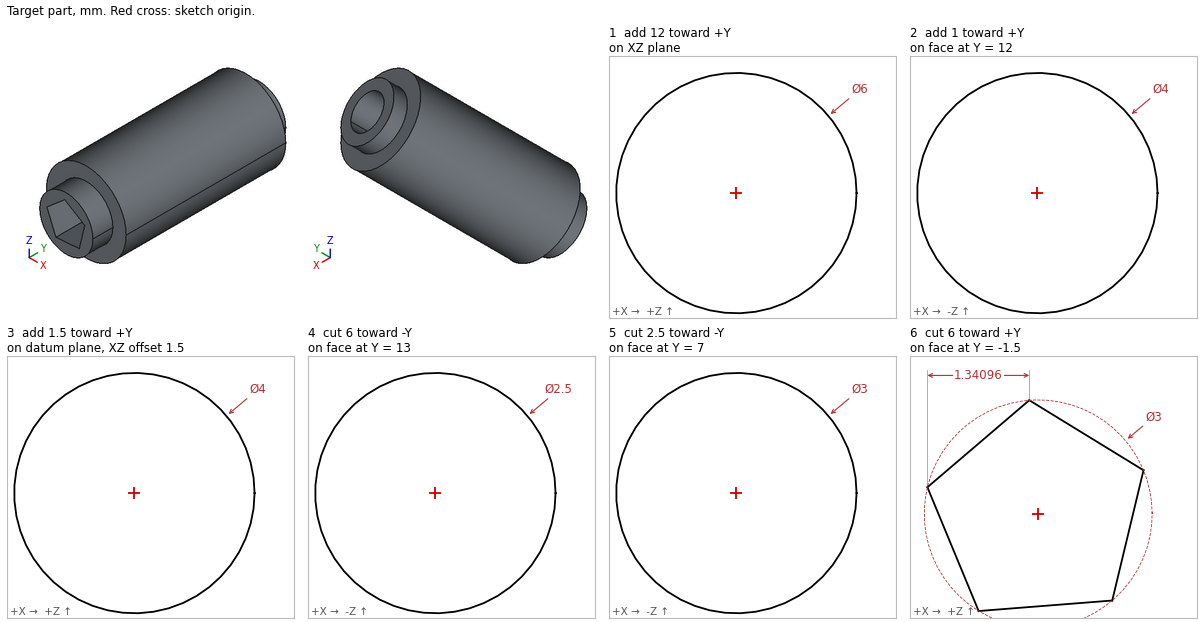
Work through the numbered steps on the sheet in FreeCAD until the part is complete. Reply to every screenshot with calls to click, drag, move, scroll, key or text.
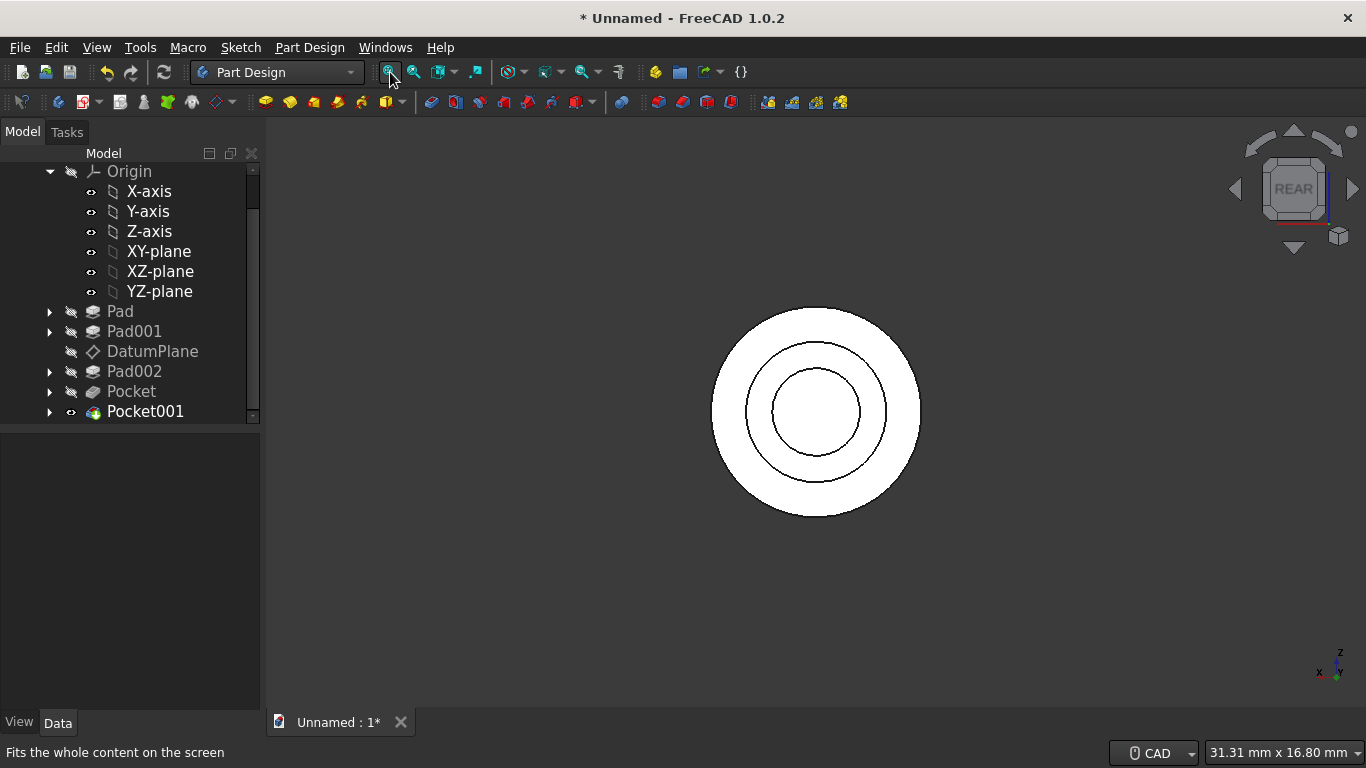
key(0)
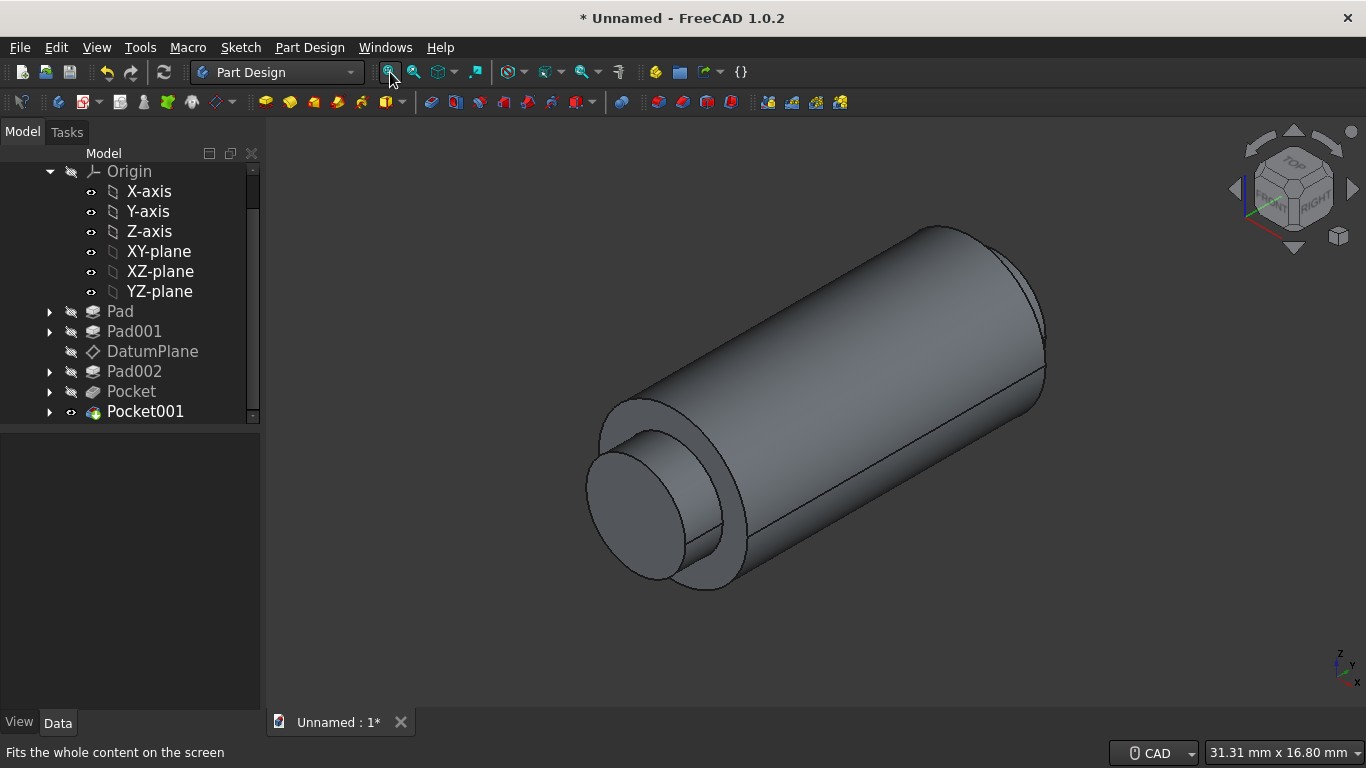
click(636, 515)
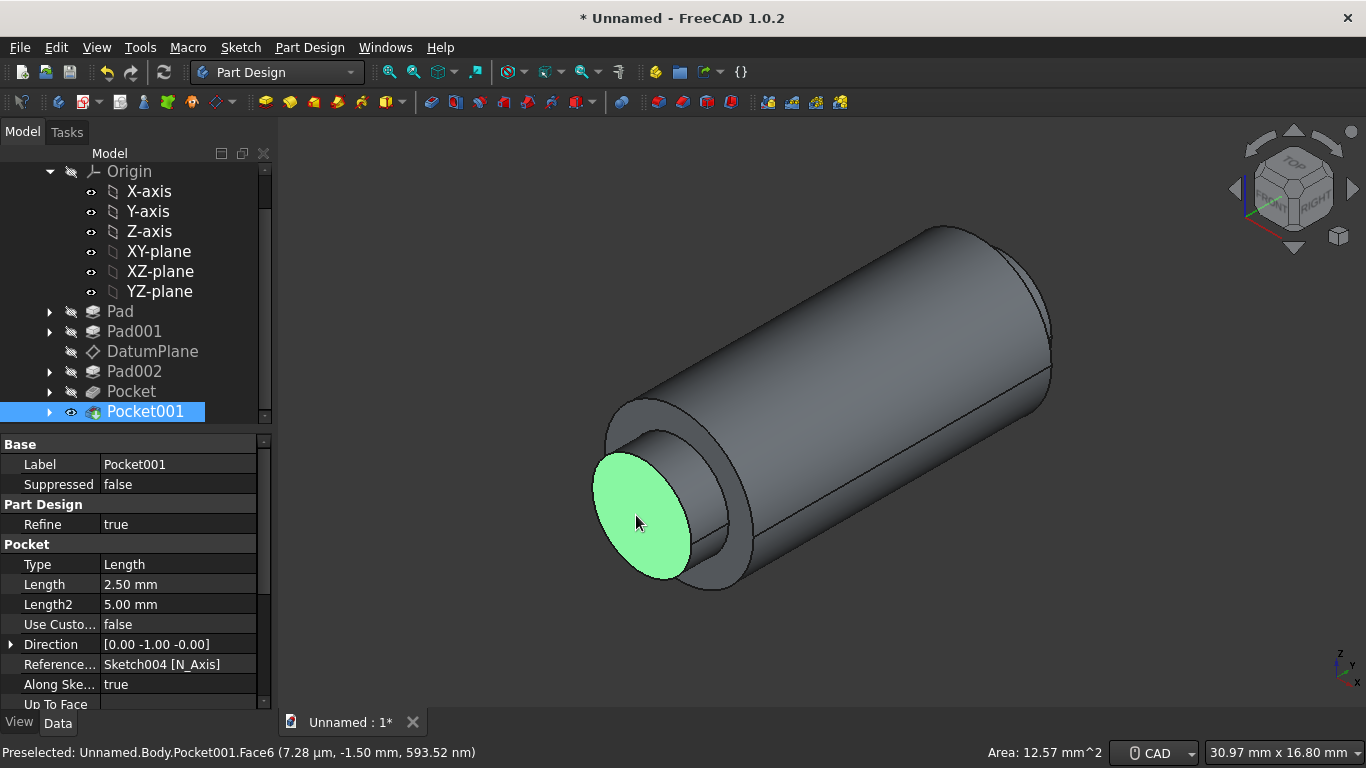
click(84, 102)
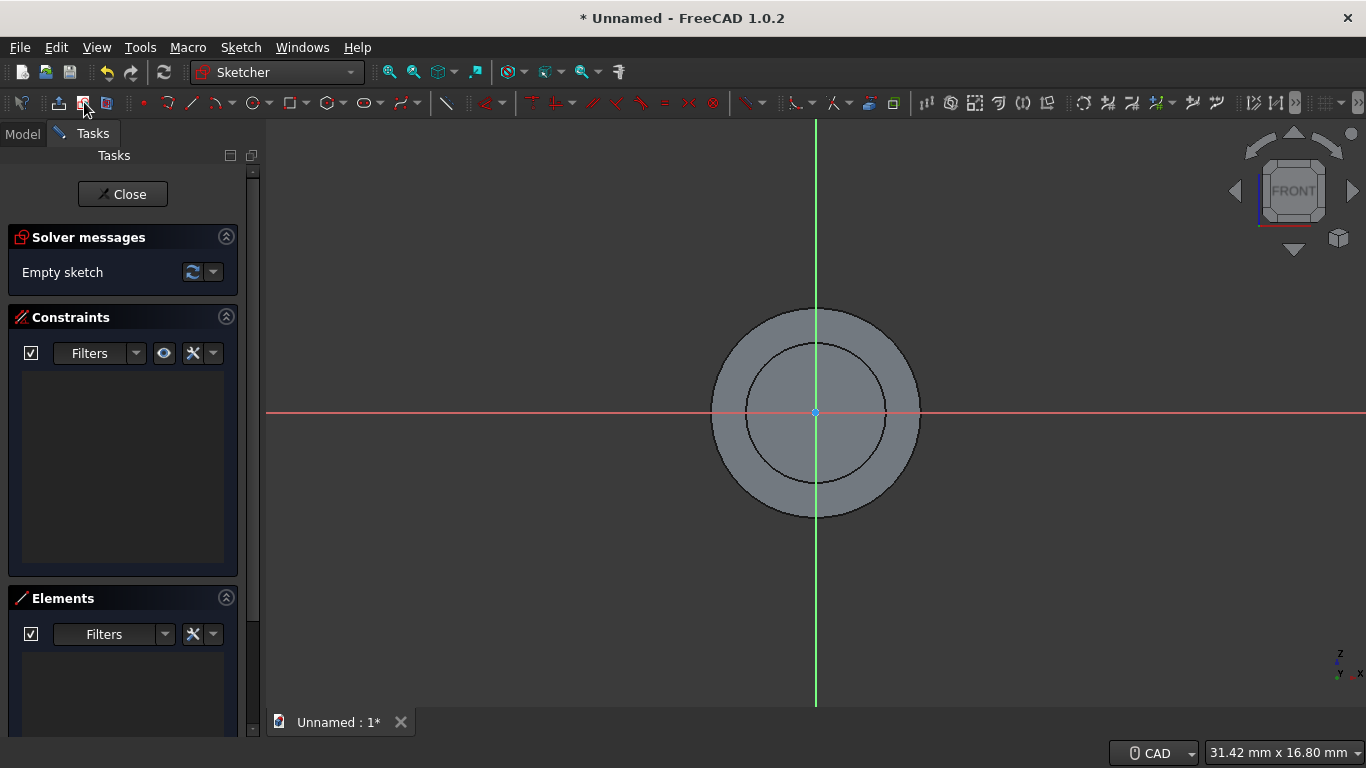
scroll(837, 408, up, 7)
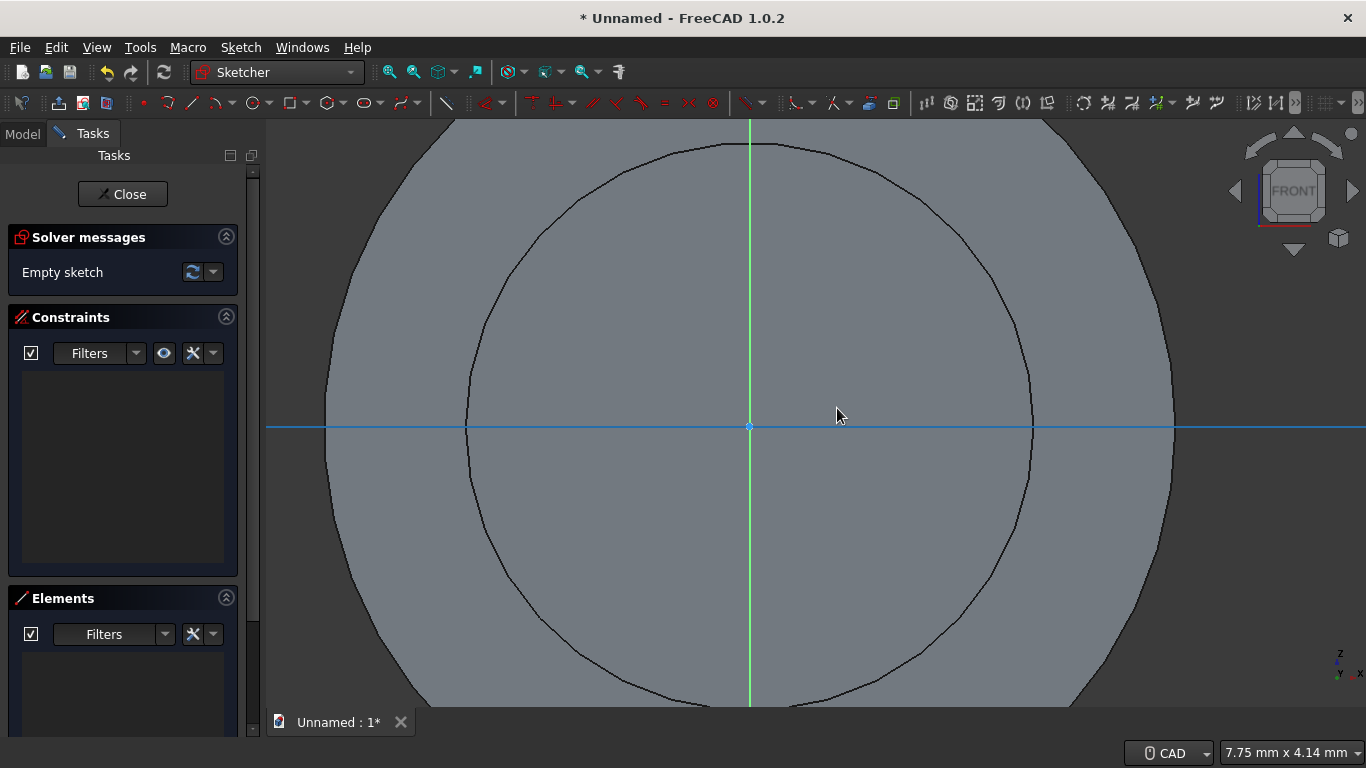
click(346, 104)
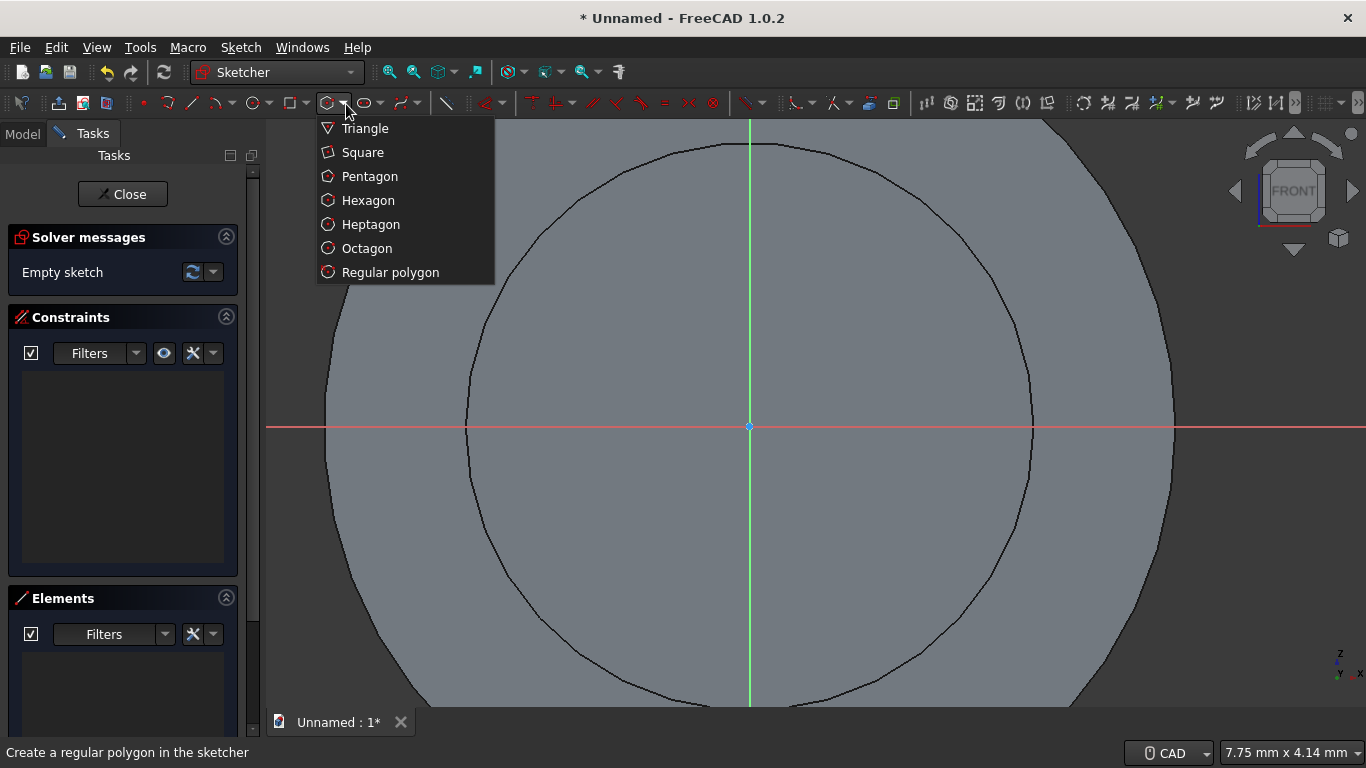
click(406, 176)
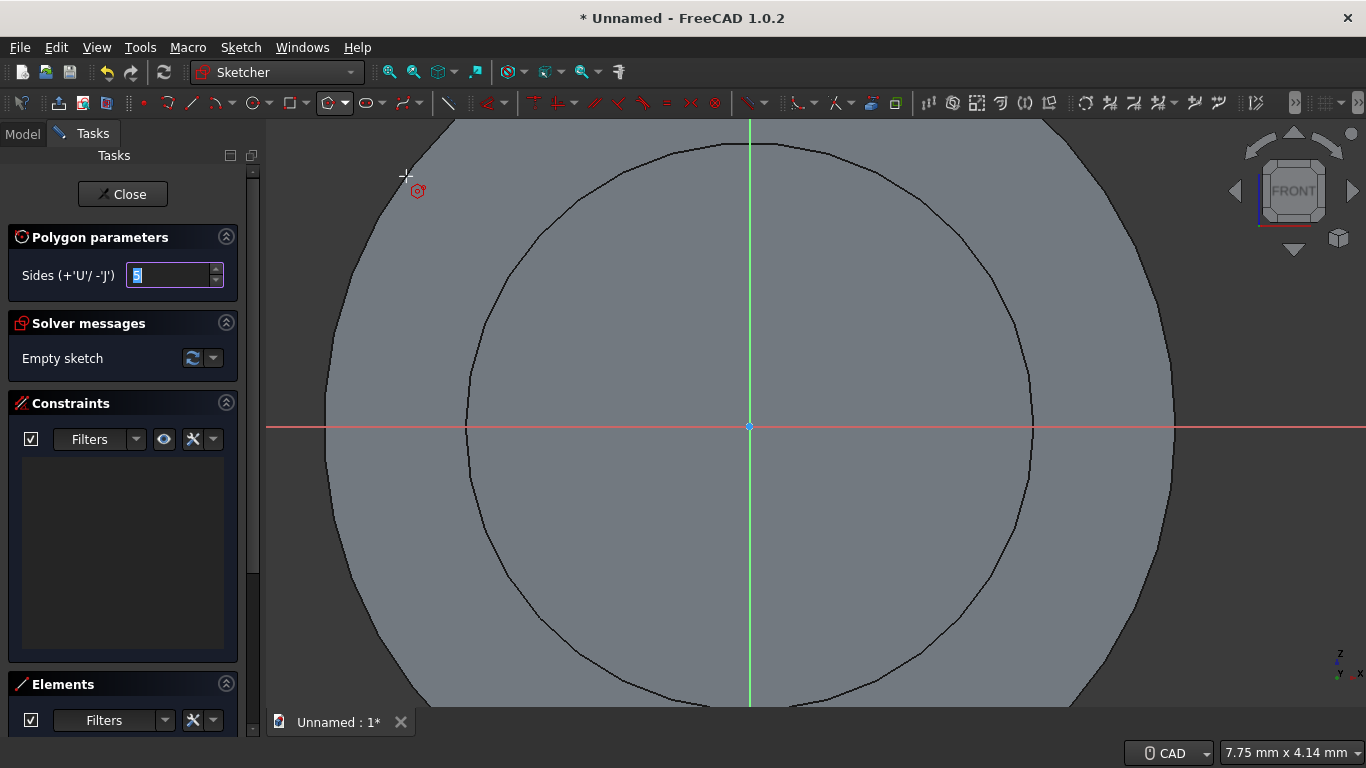
click(750, 427)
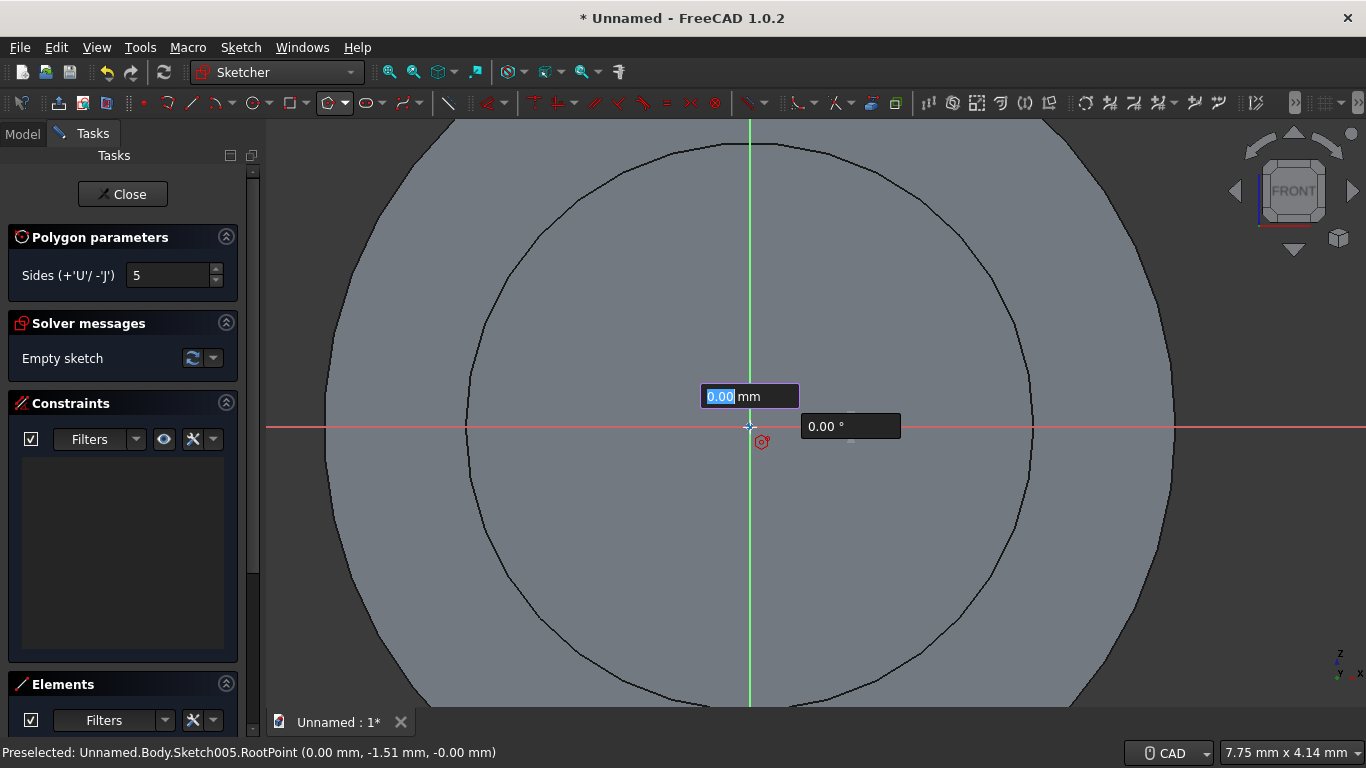
click(888, 589)
right_click(888, 589)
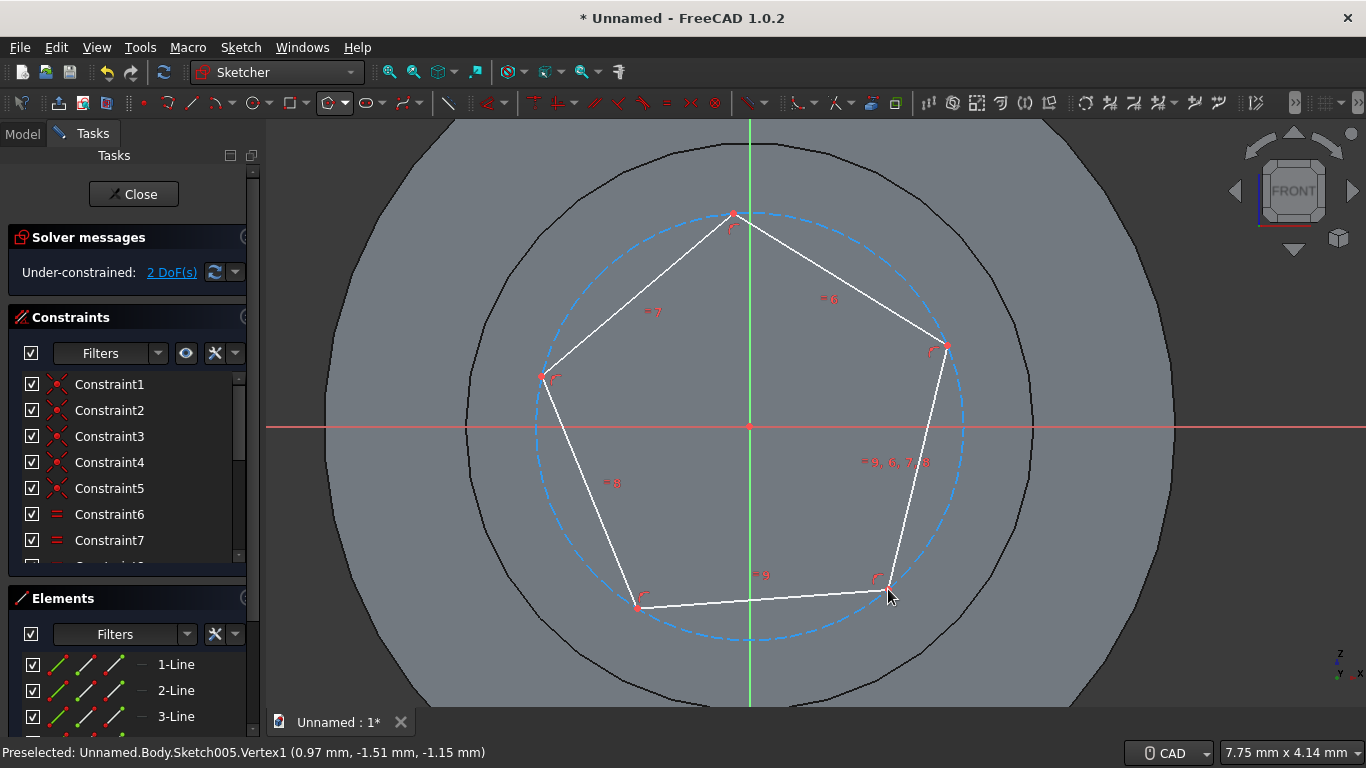
click(488, 104)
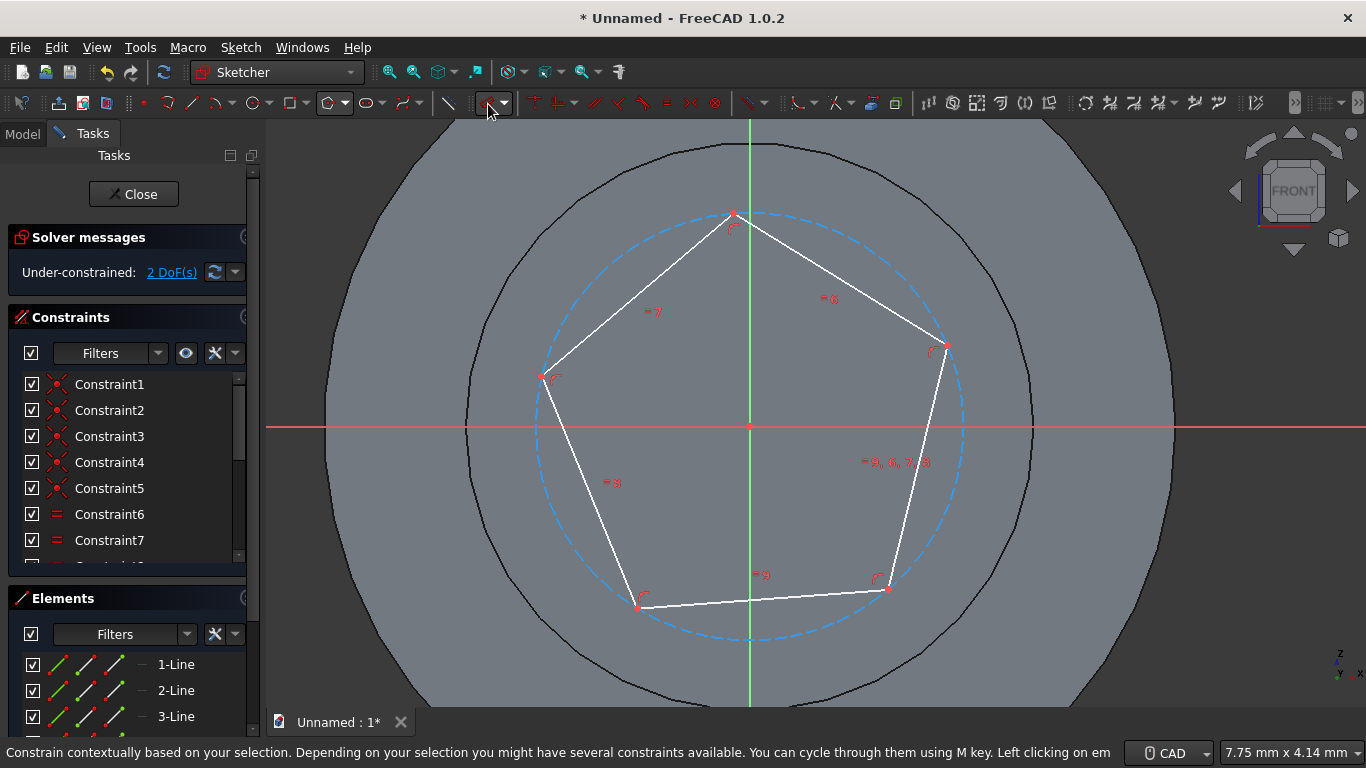
click(901, 275)
click(924, 252)